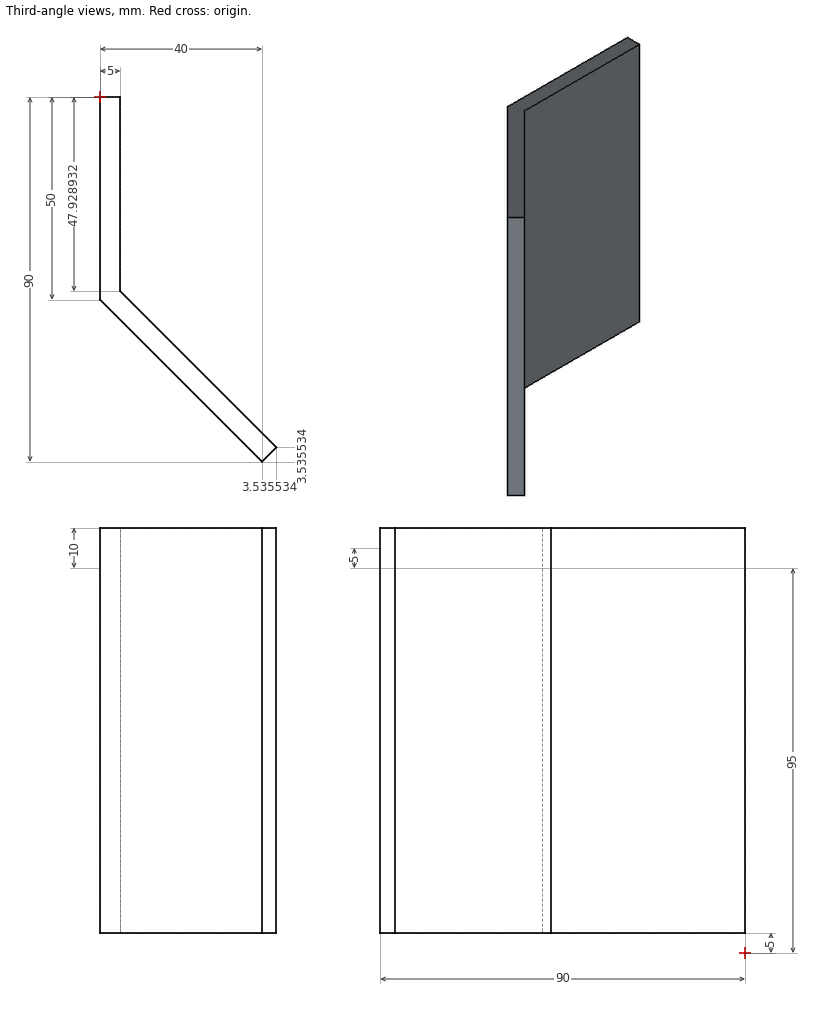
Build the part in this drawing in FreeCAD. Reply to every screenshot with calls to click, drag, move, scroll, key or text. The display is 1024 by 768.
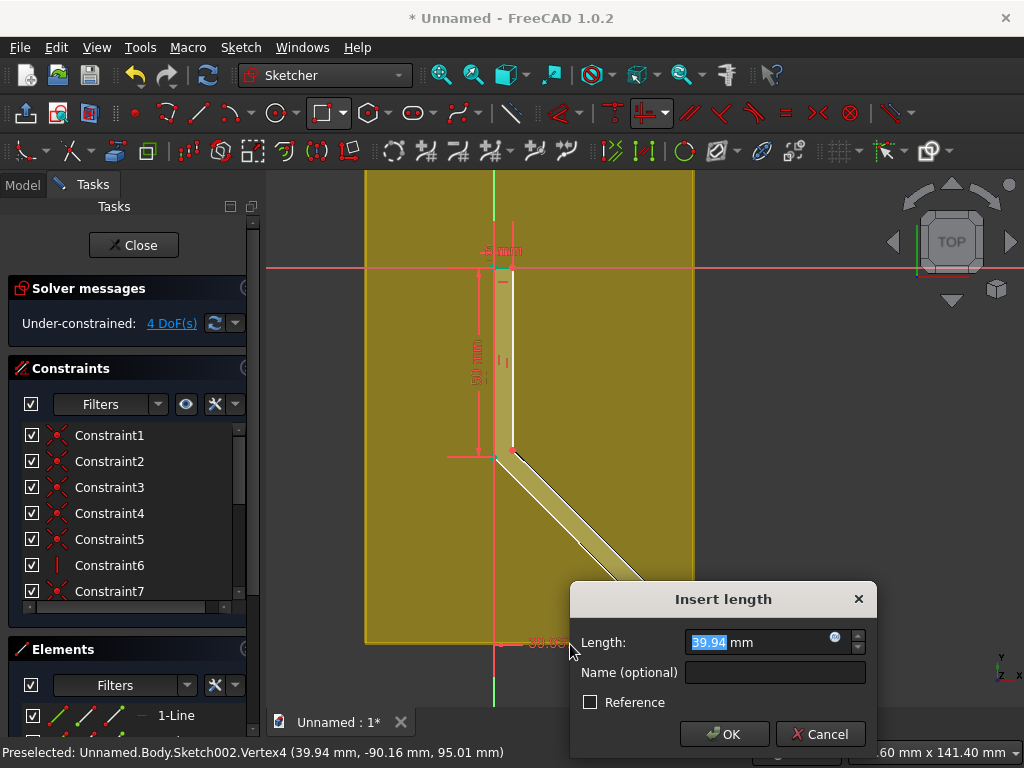
text(40)
key(Return)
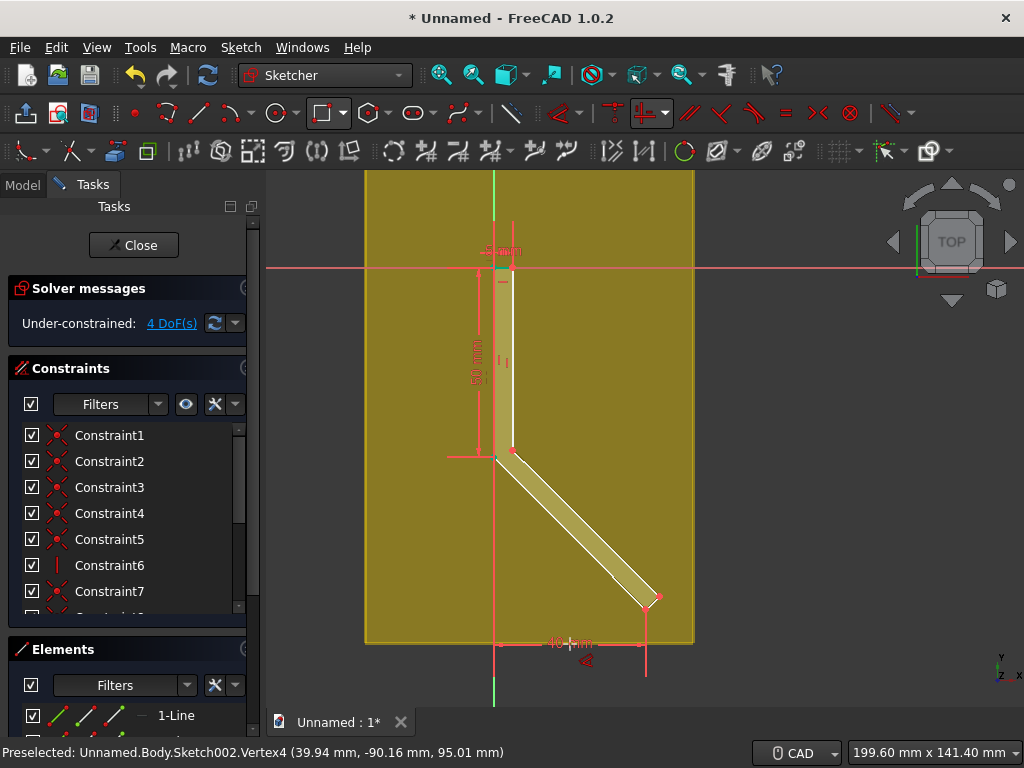
click(646, 610)
click(460, 439)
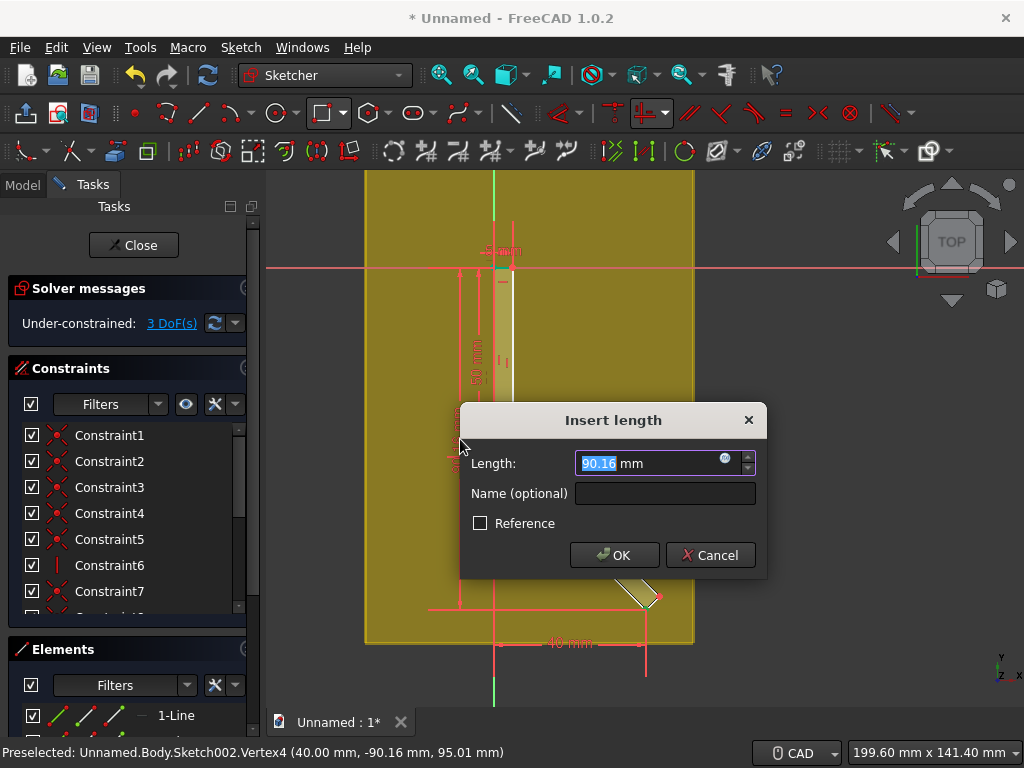
text(90)
key(Return)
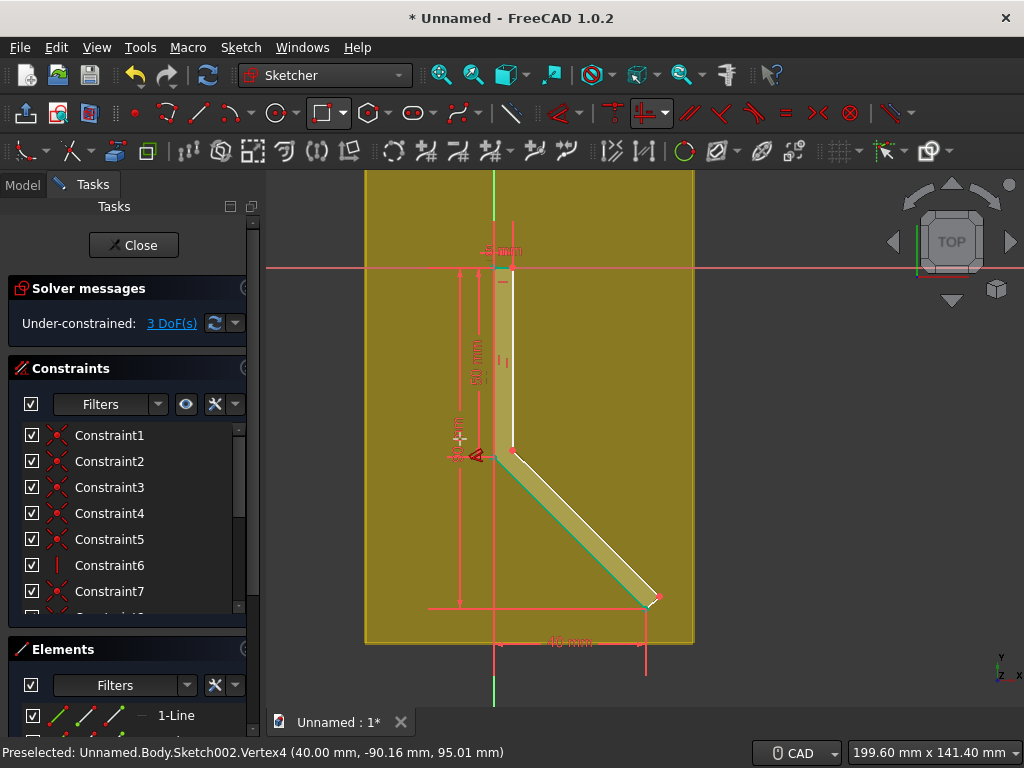
click(513, 396)
click(479, 317)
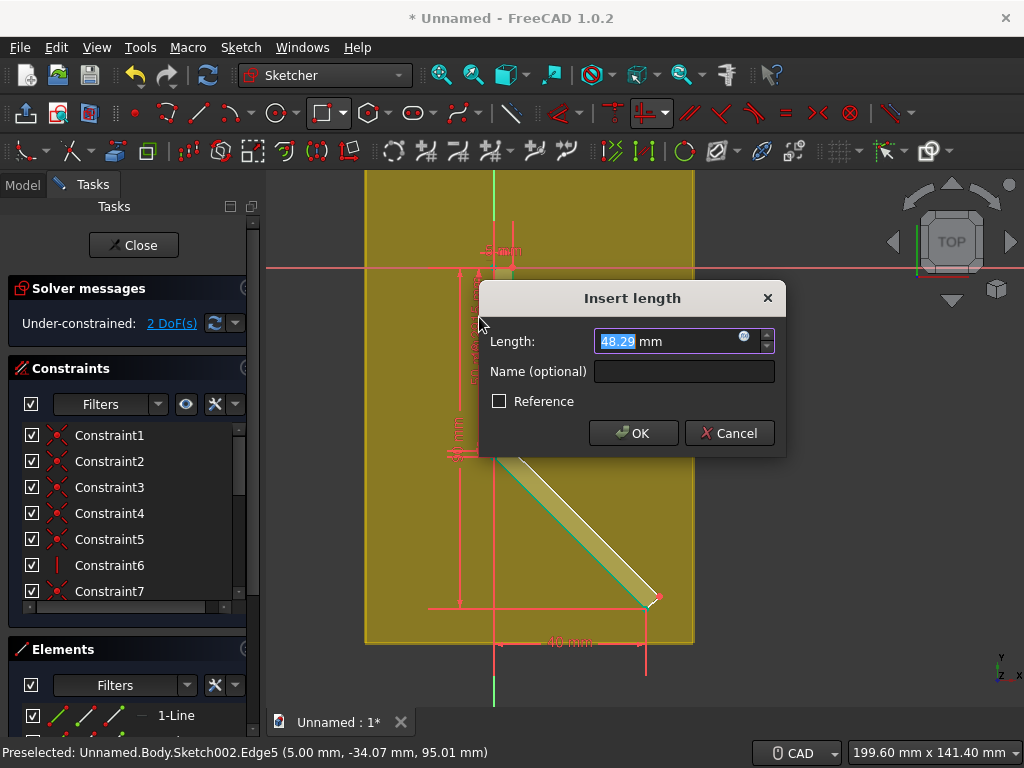
text(47.928932)
key(Return)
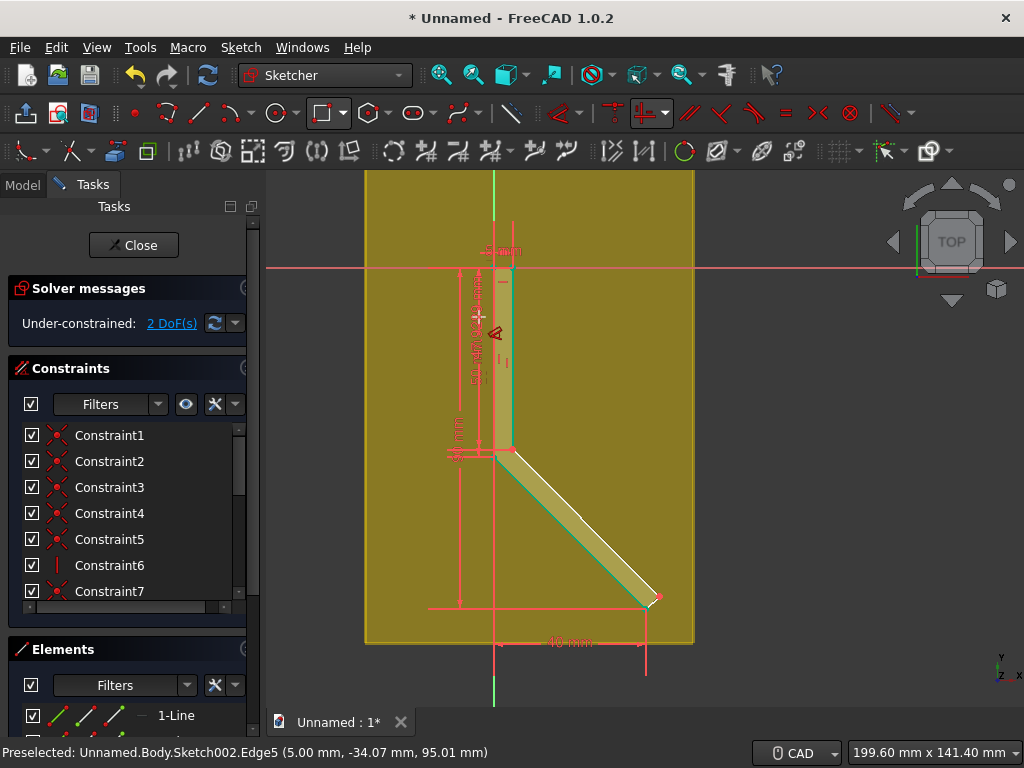
scroll(653, 603, up, 6)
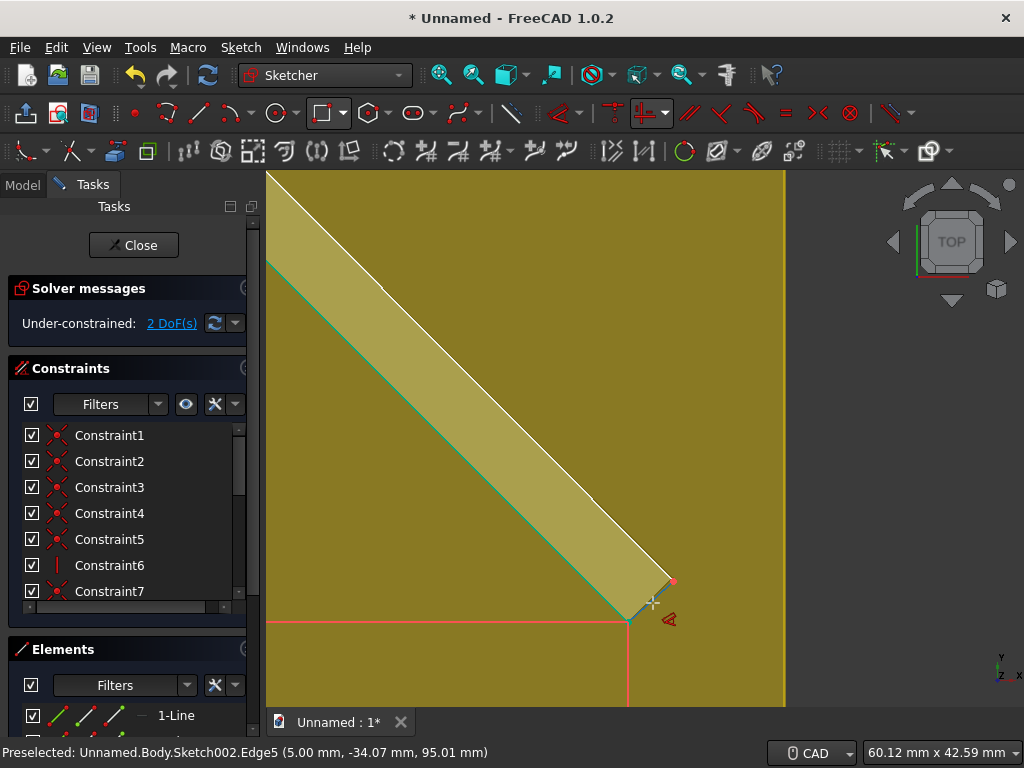
click(651, 602)
click(651, 656)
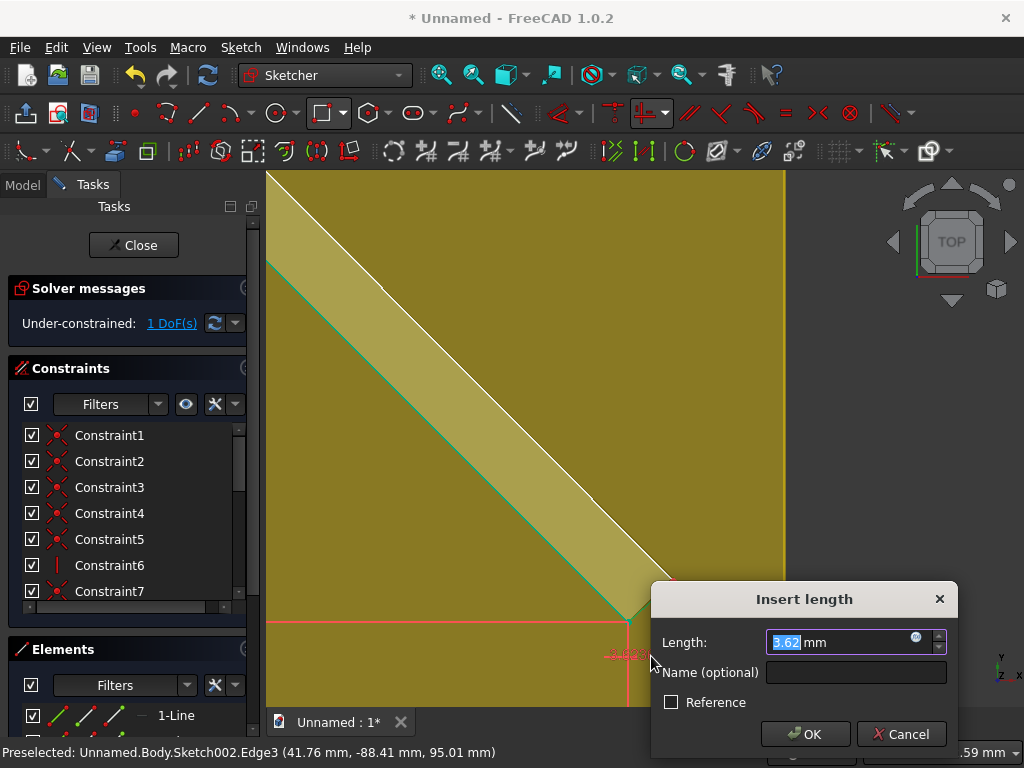
text(3.535534)
key(Return)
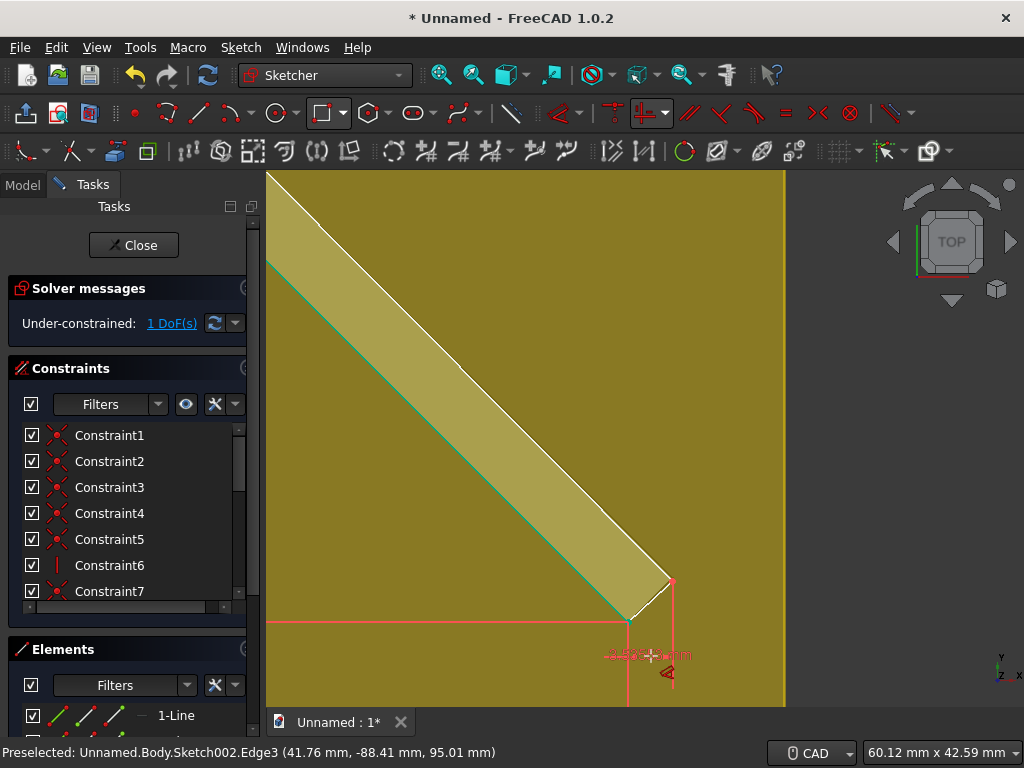
click(641, 610)
click(707, 602)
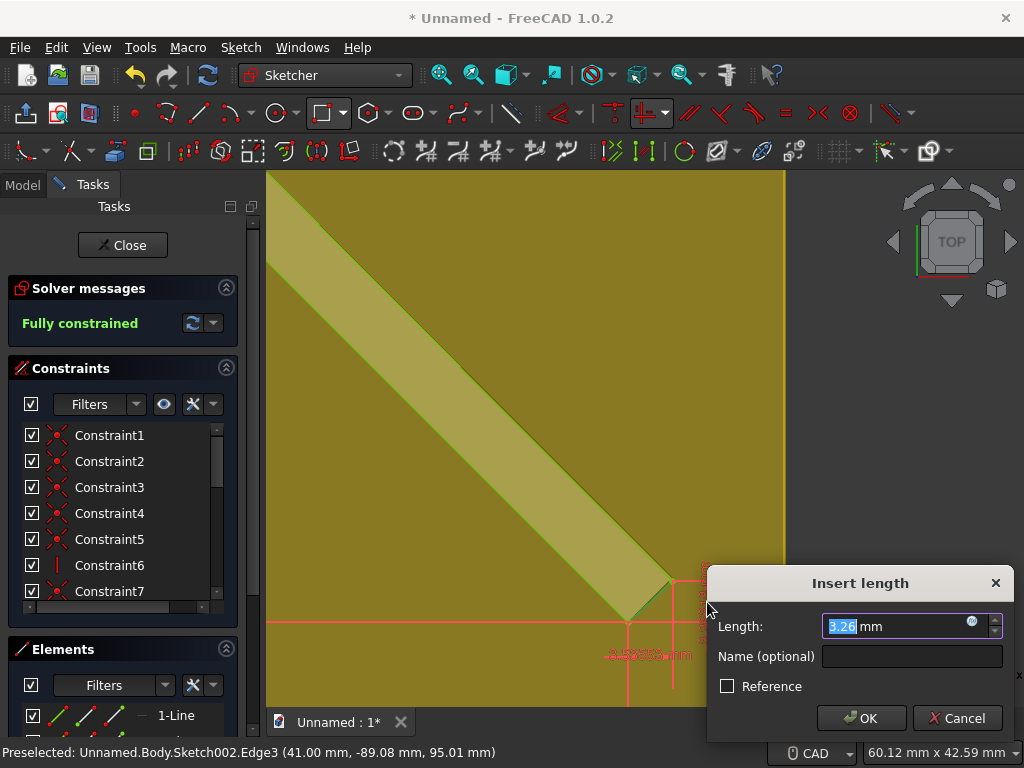
text(3.535534)
key(Return)
key(Escape)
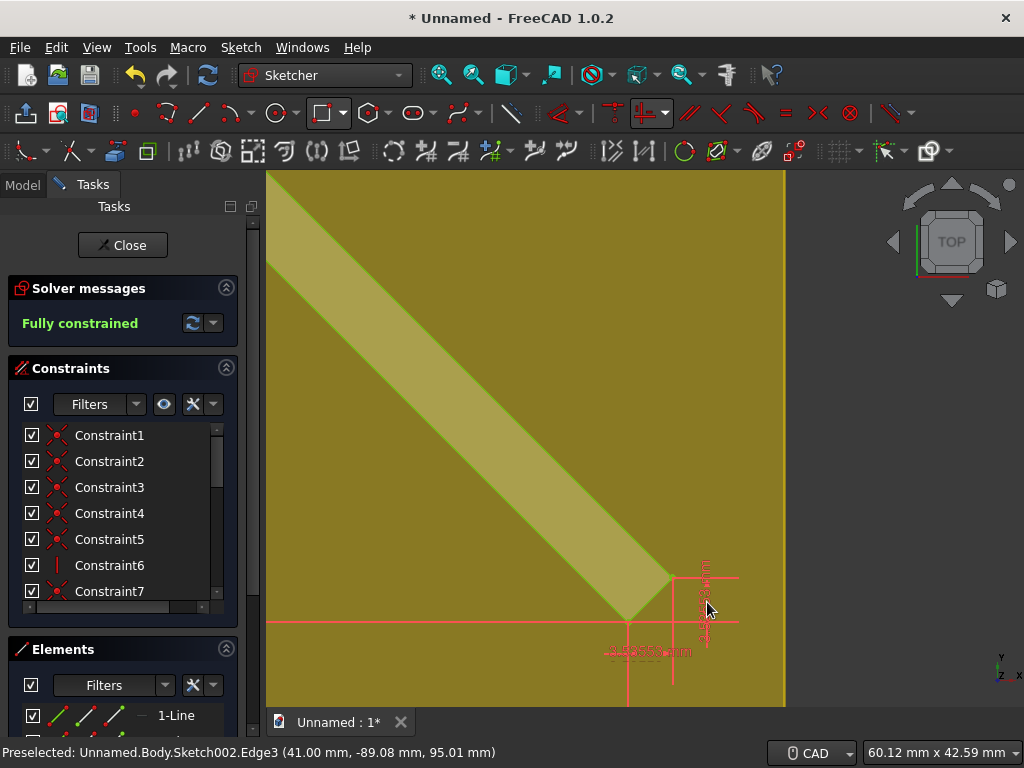
click(123, 245)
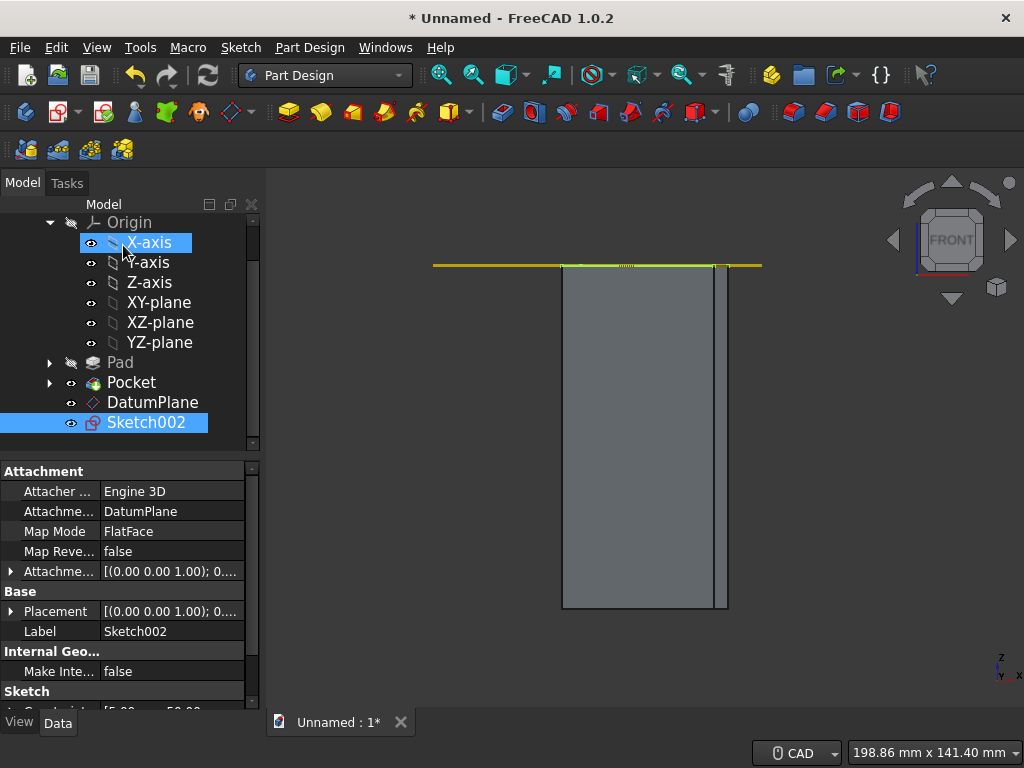
click(290, 112)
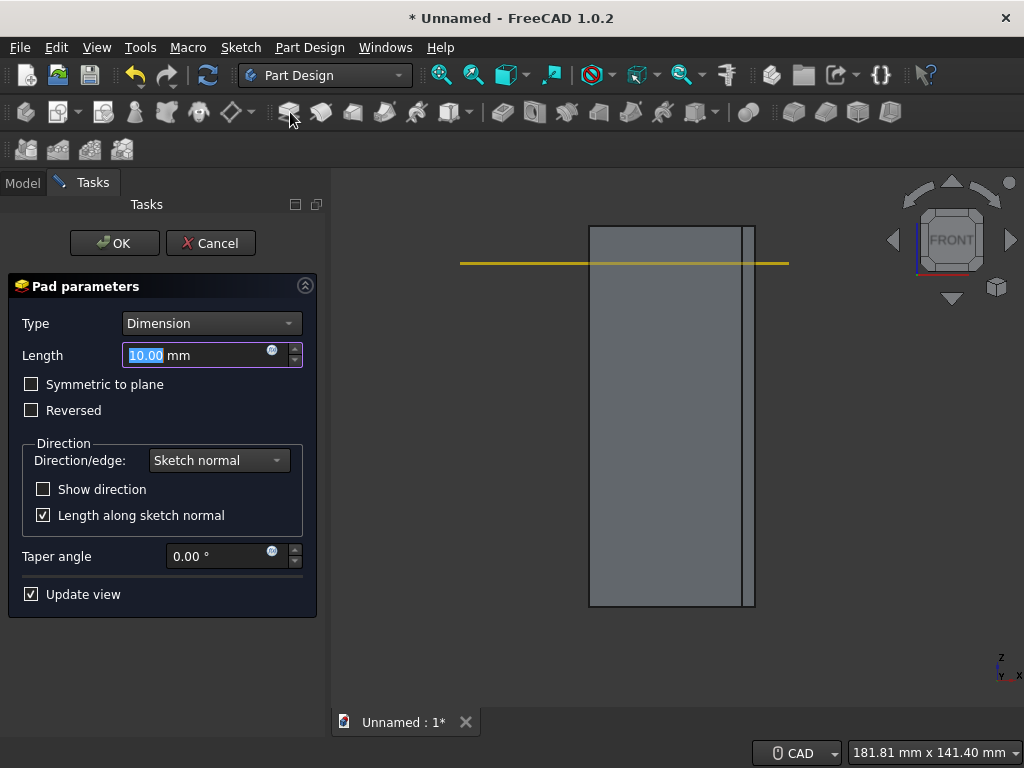
text(10)
key(Tab)